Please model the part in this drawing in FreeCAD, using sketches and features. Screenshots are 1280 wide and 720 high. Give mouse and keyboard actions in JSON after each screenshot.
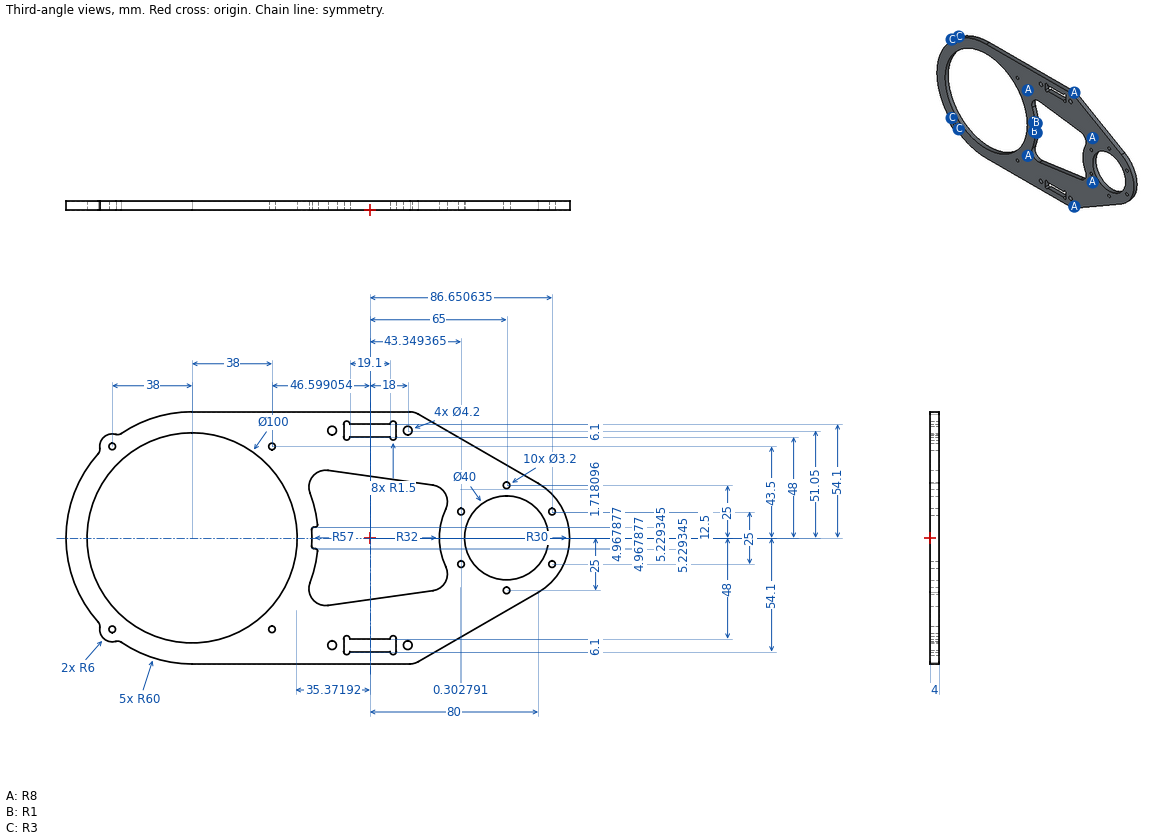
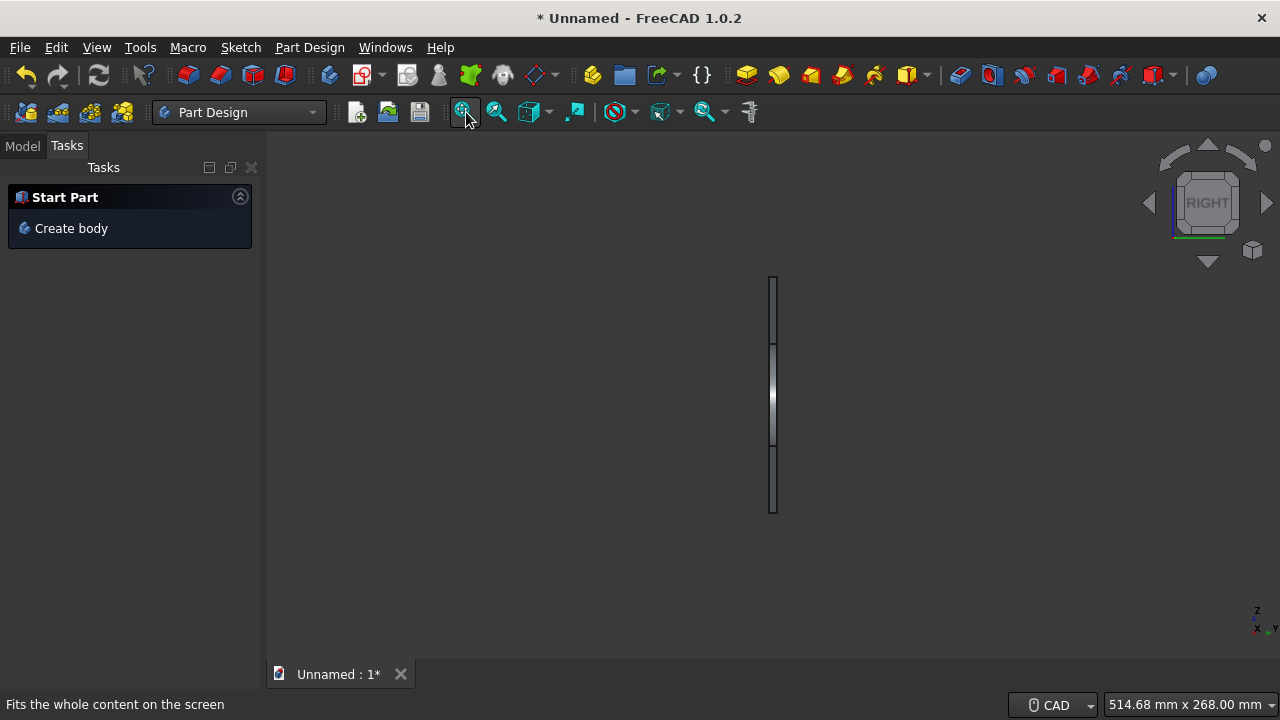
{"action": "scroll", "coordinate": [773, 462], "scroll_direction": "up", "scroll_amount": 9}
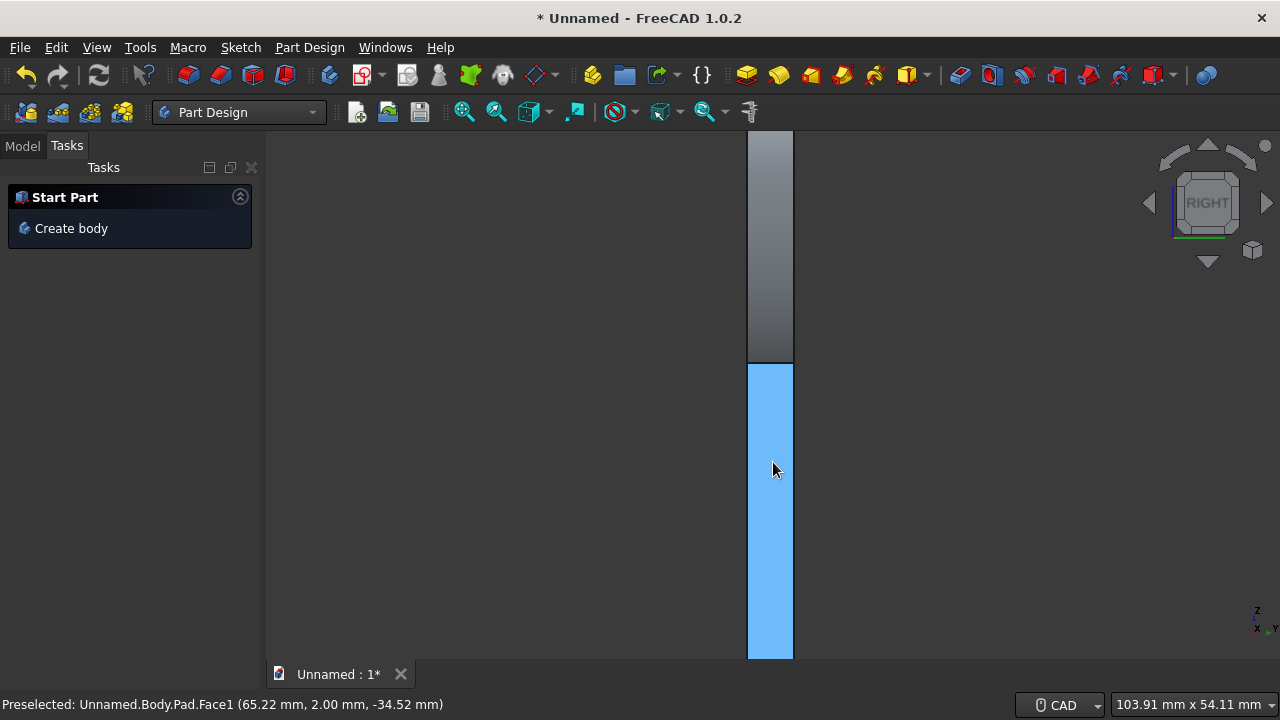
{"action": "left_click", "coordinate": [466, 112]}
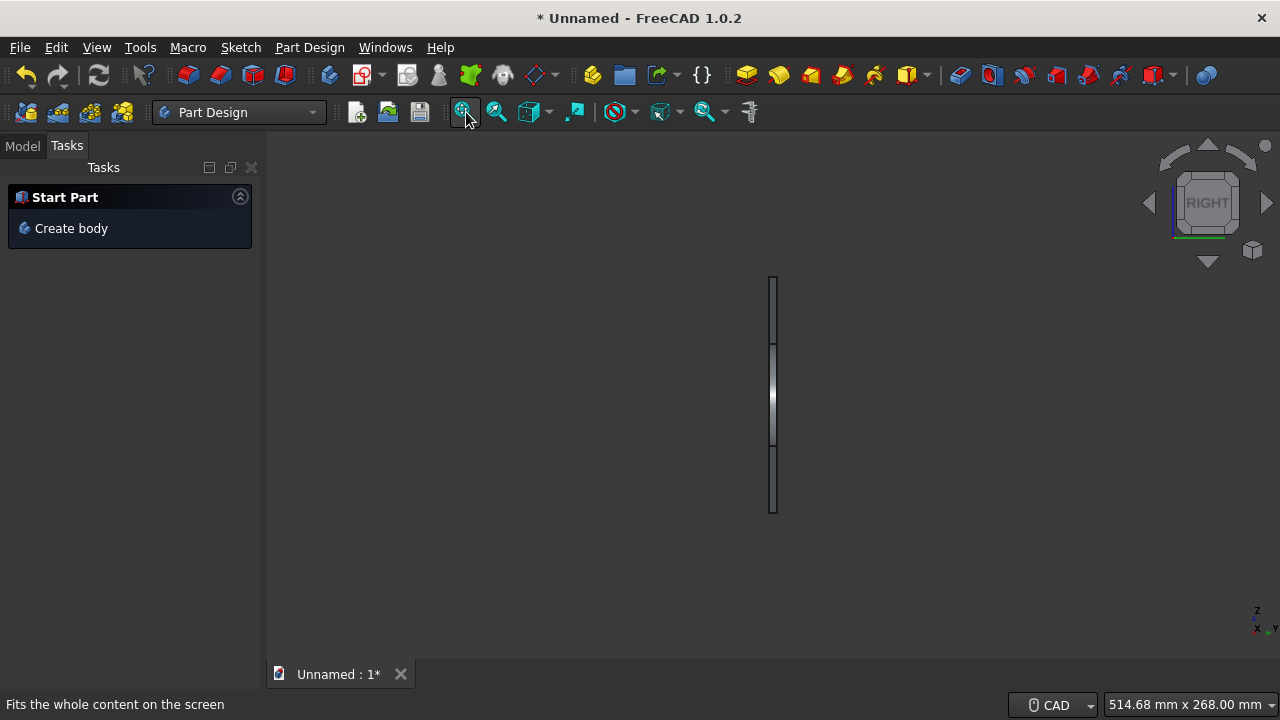
{"action": "key", "text": "5"}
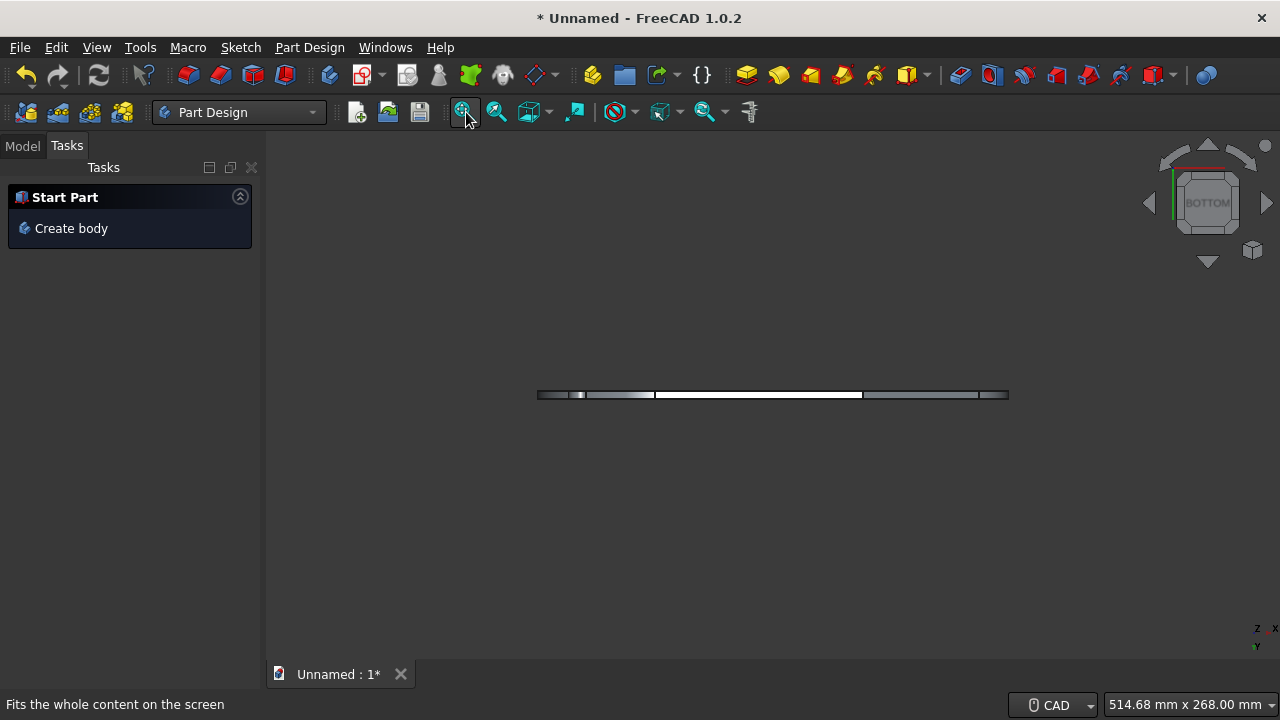
{"action": "scroll", "coordinate": [752, 394], "scroll_direction": "up", "scroll_amount": 9}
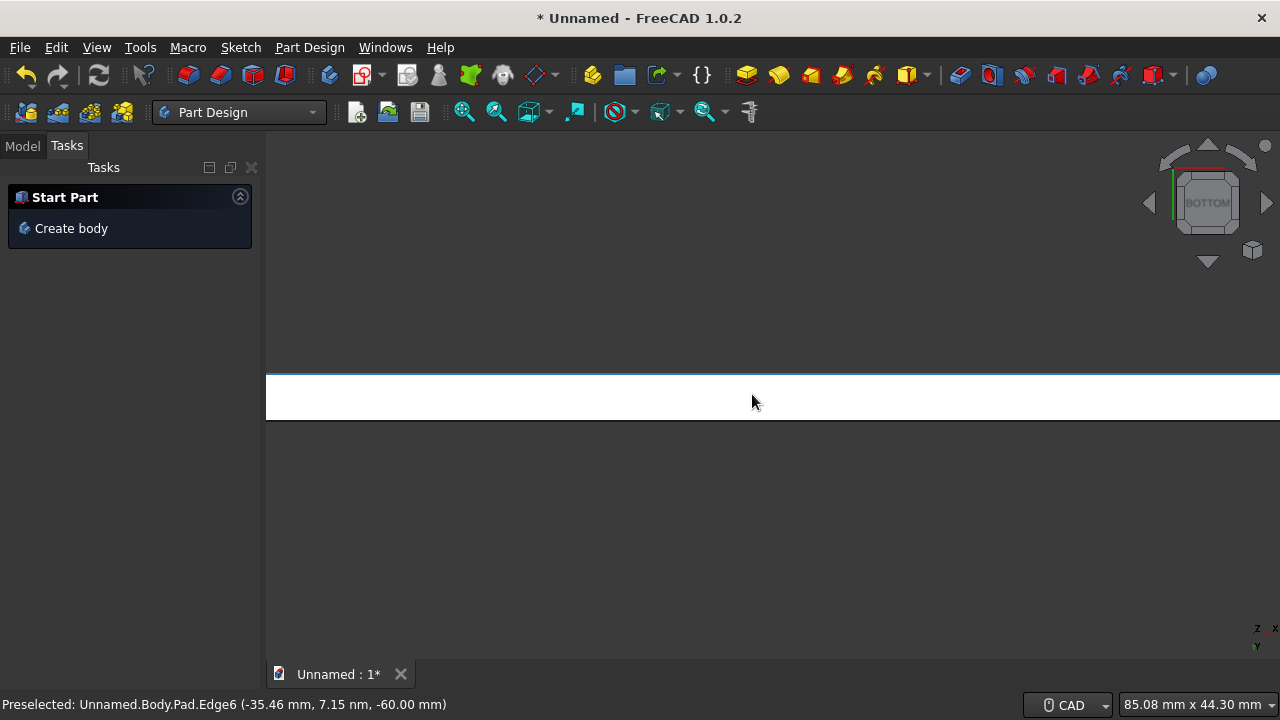
{"action": "left_click", "coordinate": [466, 112]}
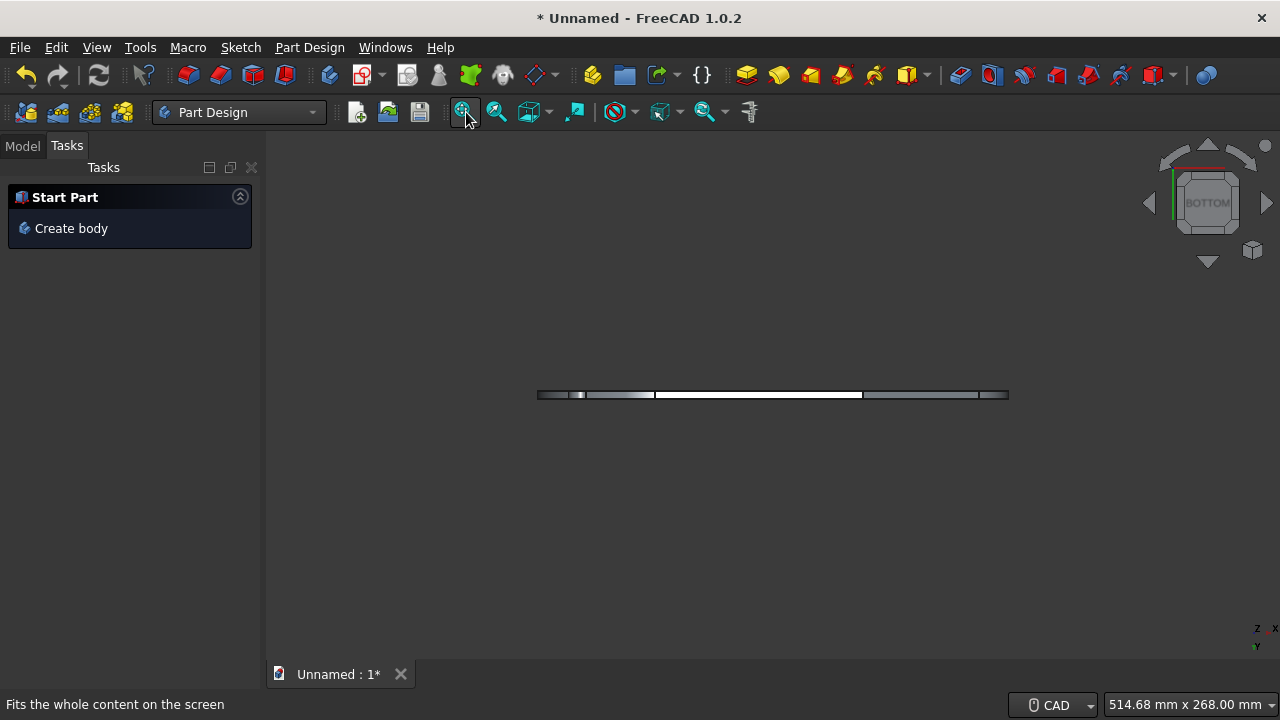
{"action": "key", "text": "4"}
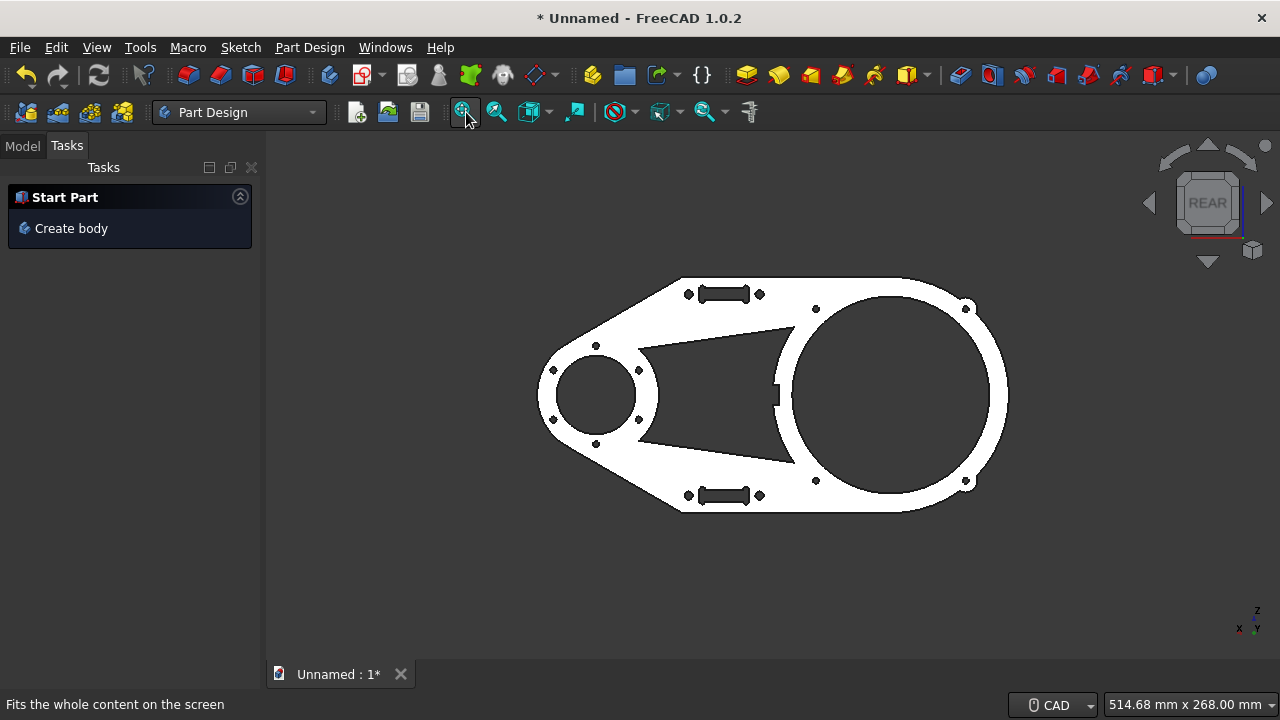
{"action": "scroll", "coordinate": [794, 462], "scroll_direction": "up", "scroll_amount": 9}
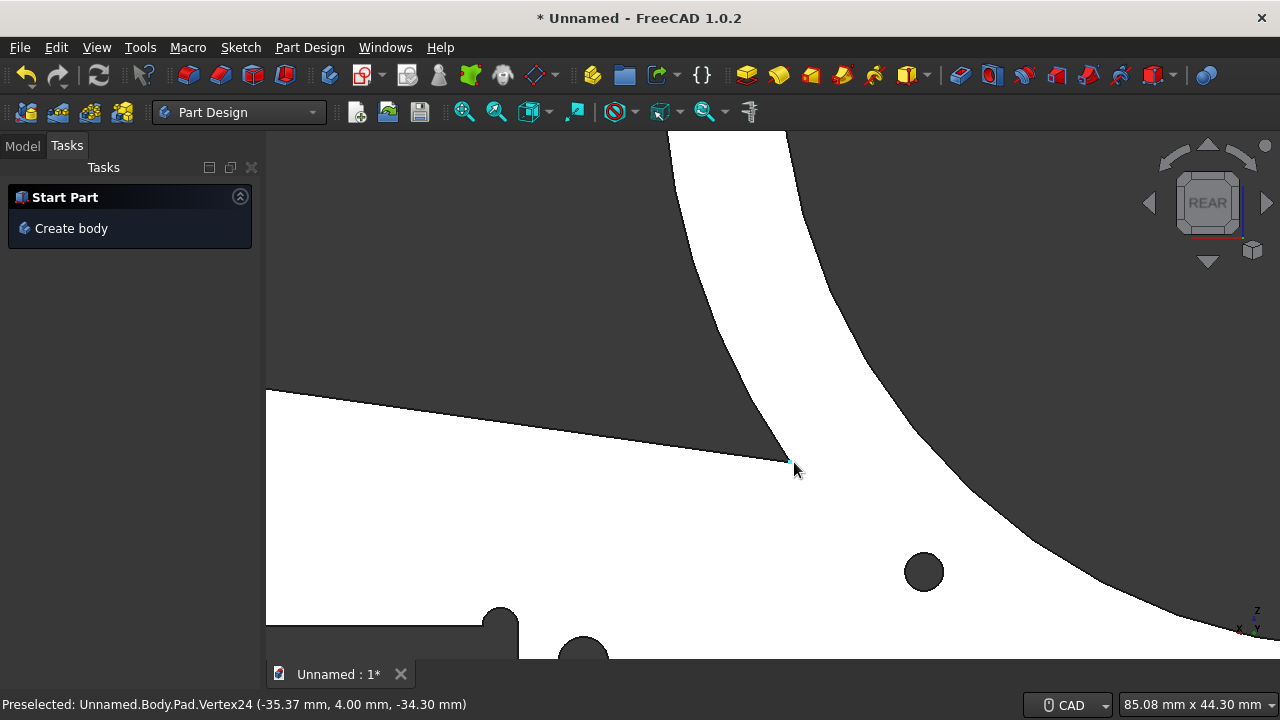
{"action": "key", "text": "v f"}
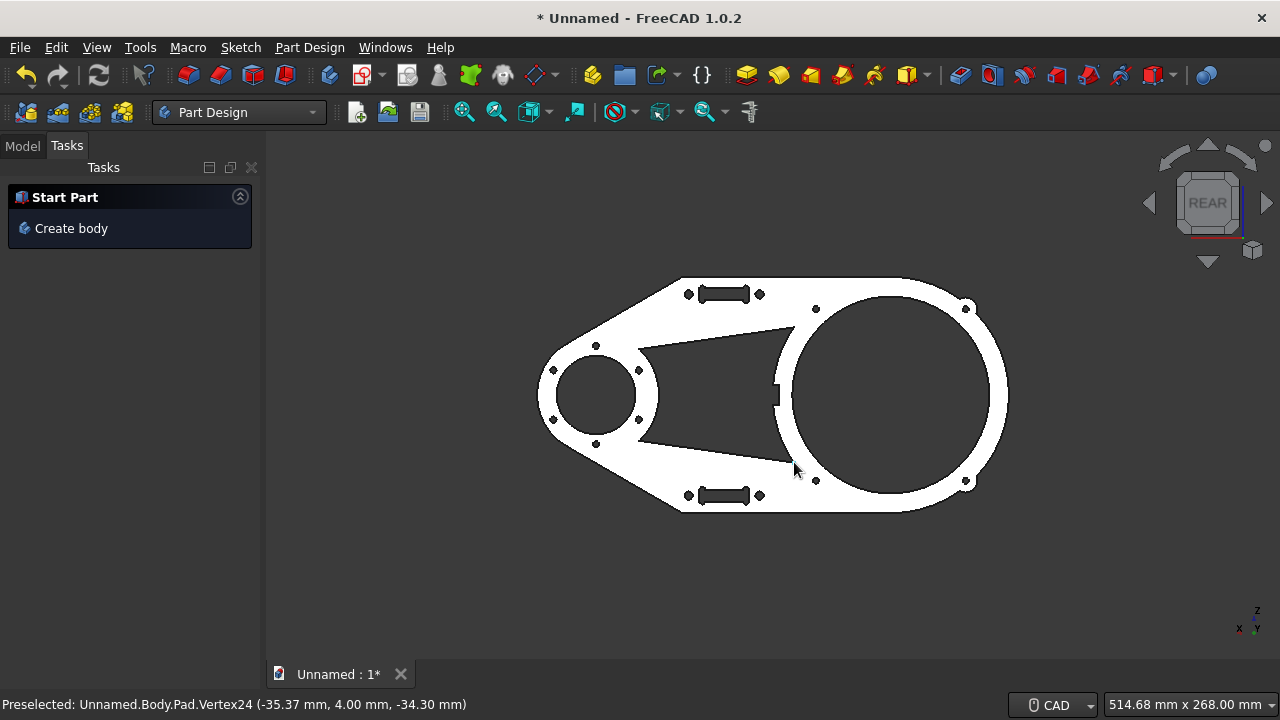
{"action": "key", "text": "6"}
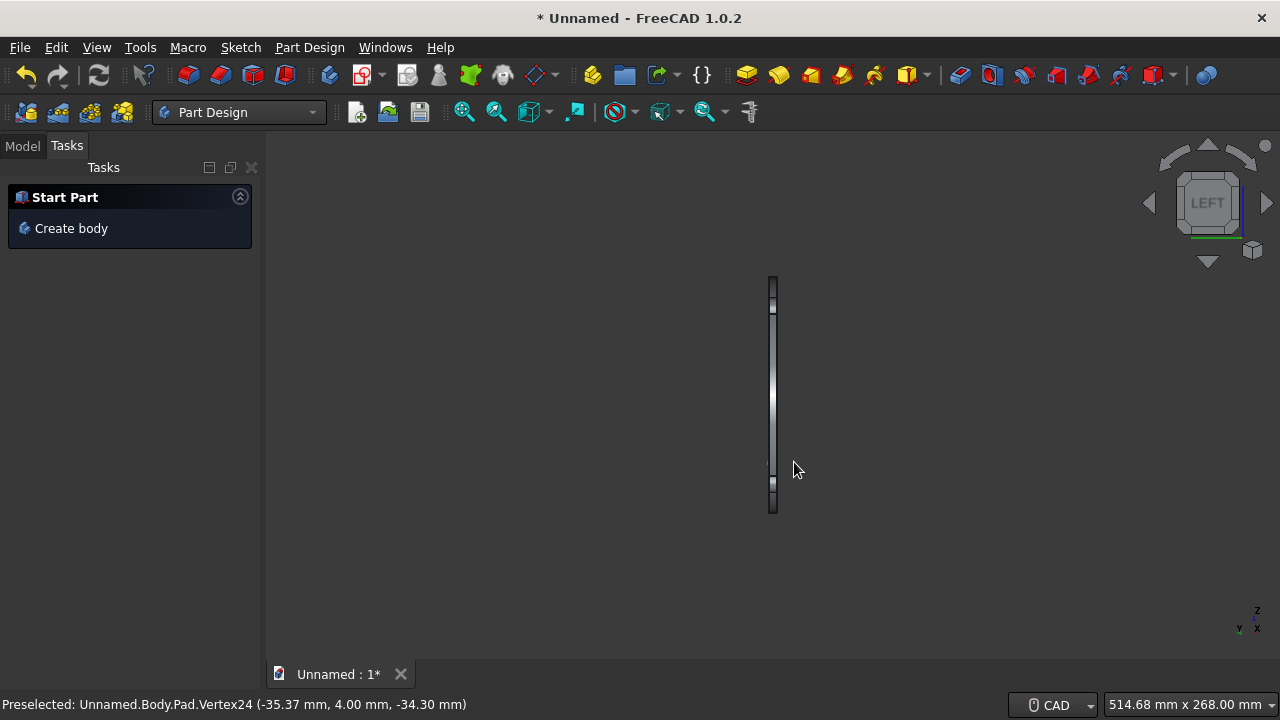
{"action": "left_click", "coordinate": [466, 112]}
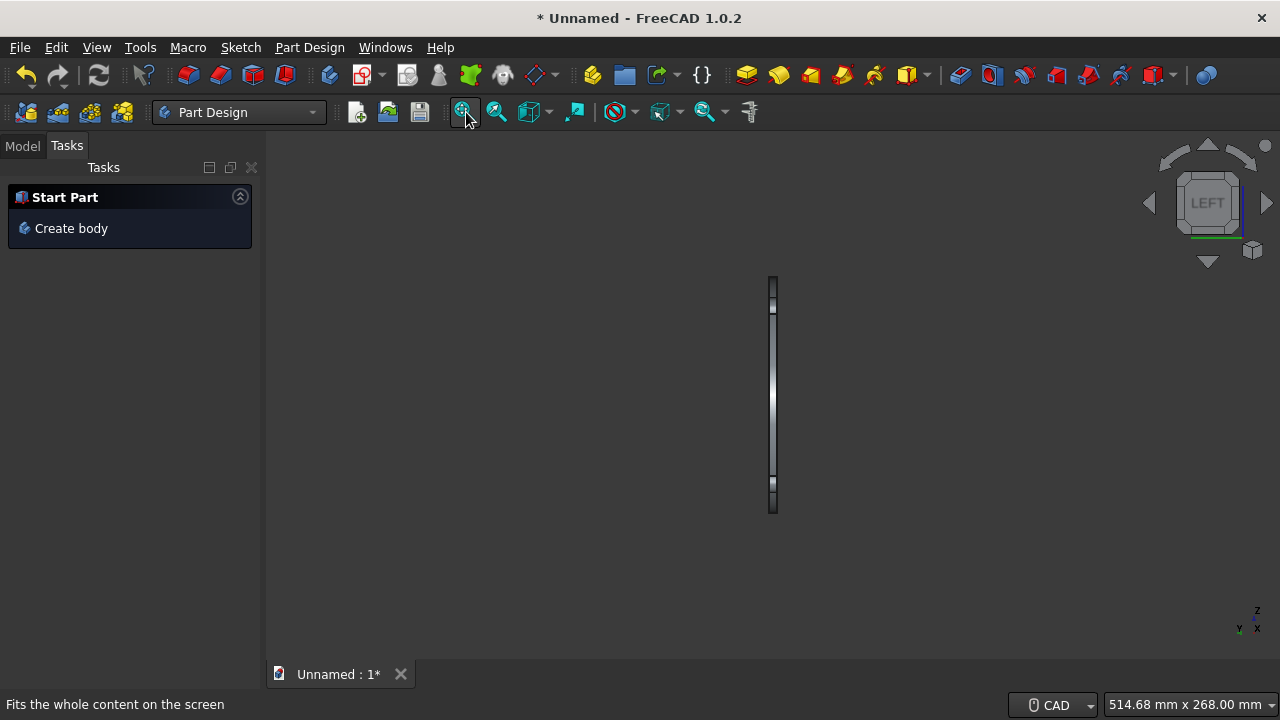
{"action": "scroll", "coordinate": [773, 462], "scroll_direction": "up", "scroll_amount": 9}